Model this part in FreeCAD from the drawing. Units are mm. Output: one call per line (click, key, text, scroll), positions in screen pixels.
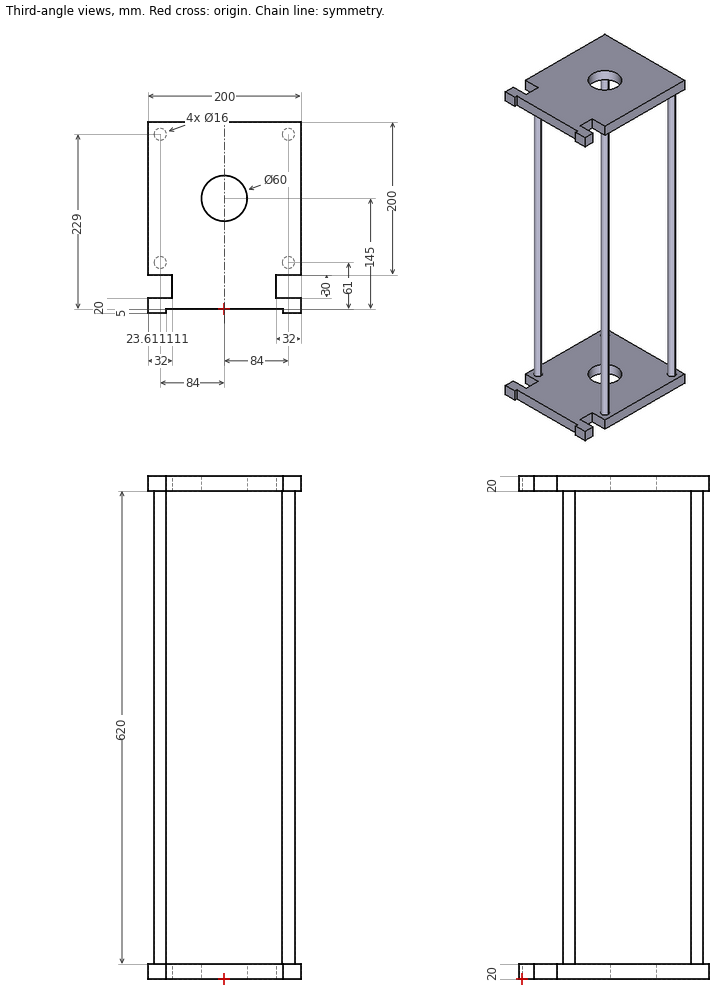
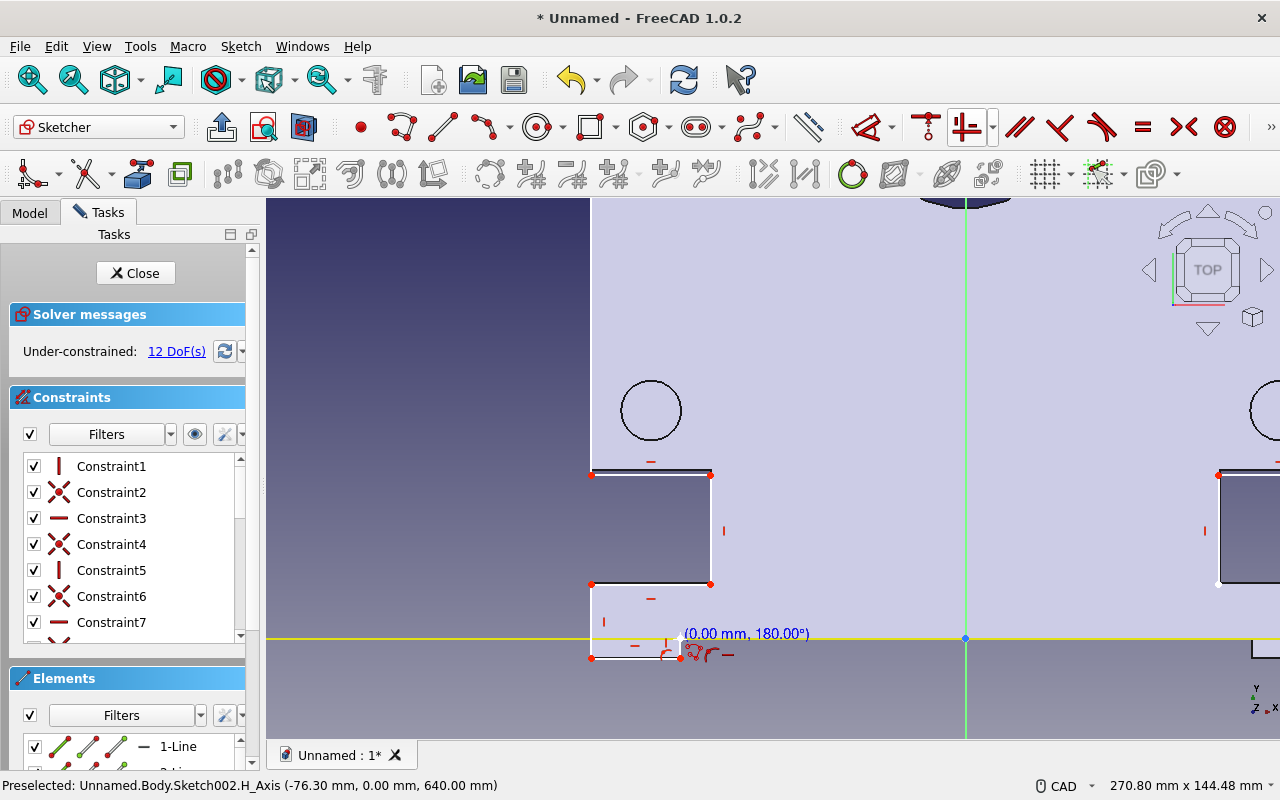
scroll(552, 631, down, 5)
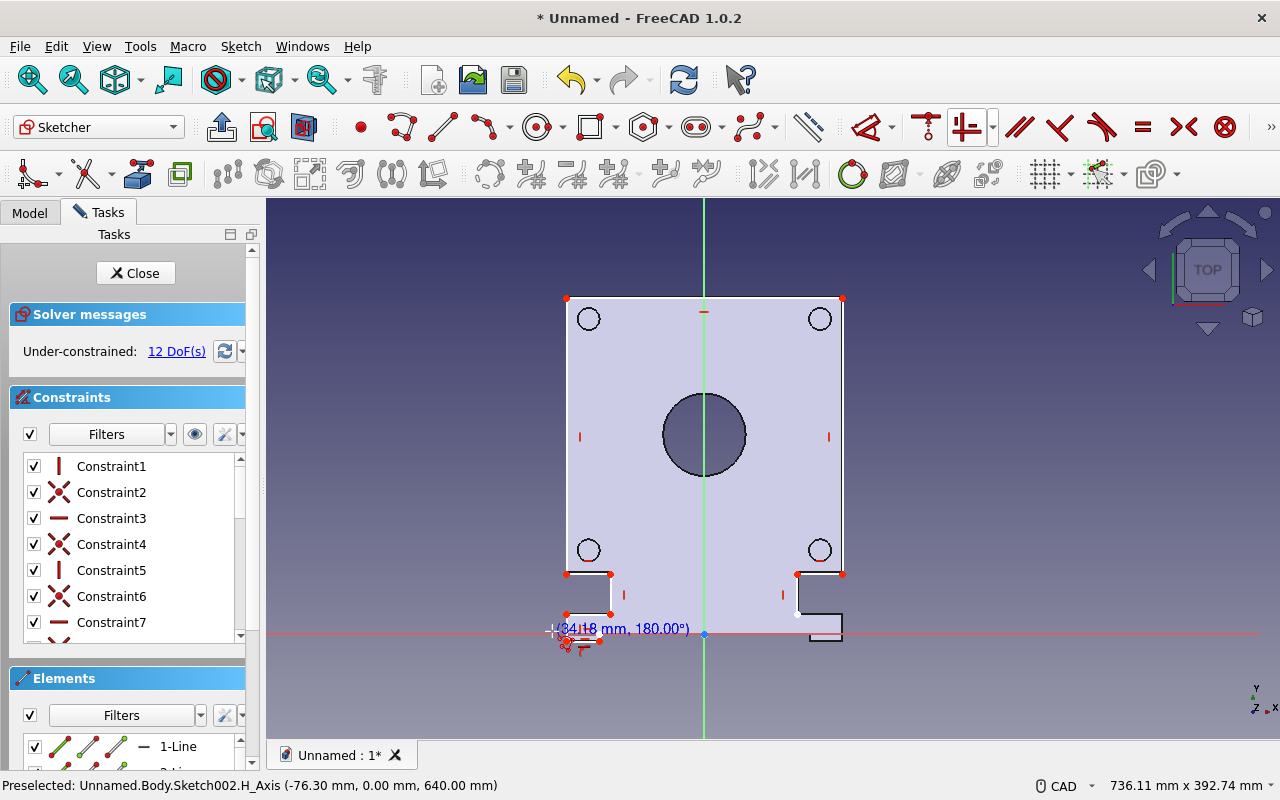
click(810, 625)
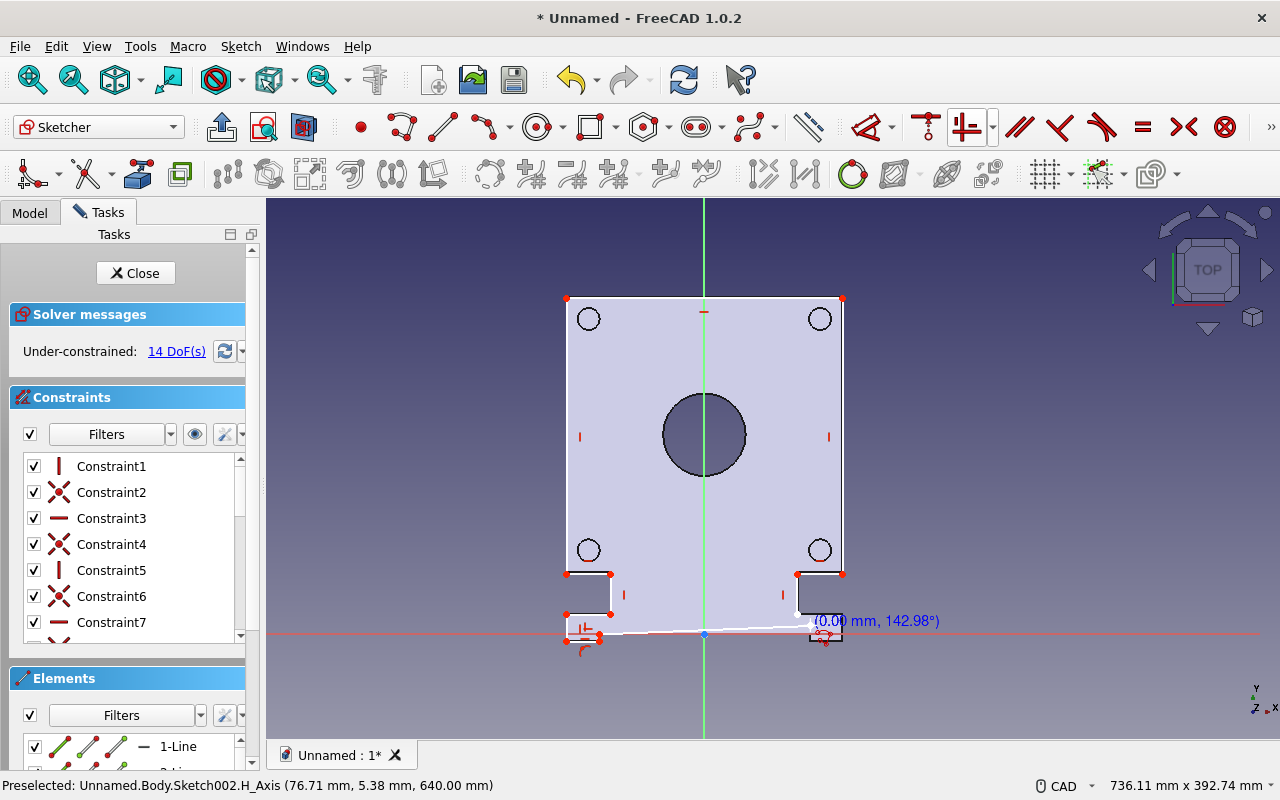
scroll(810, 641, up, 5)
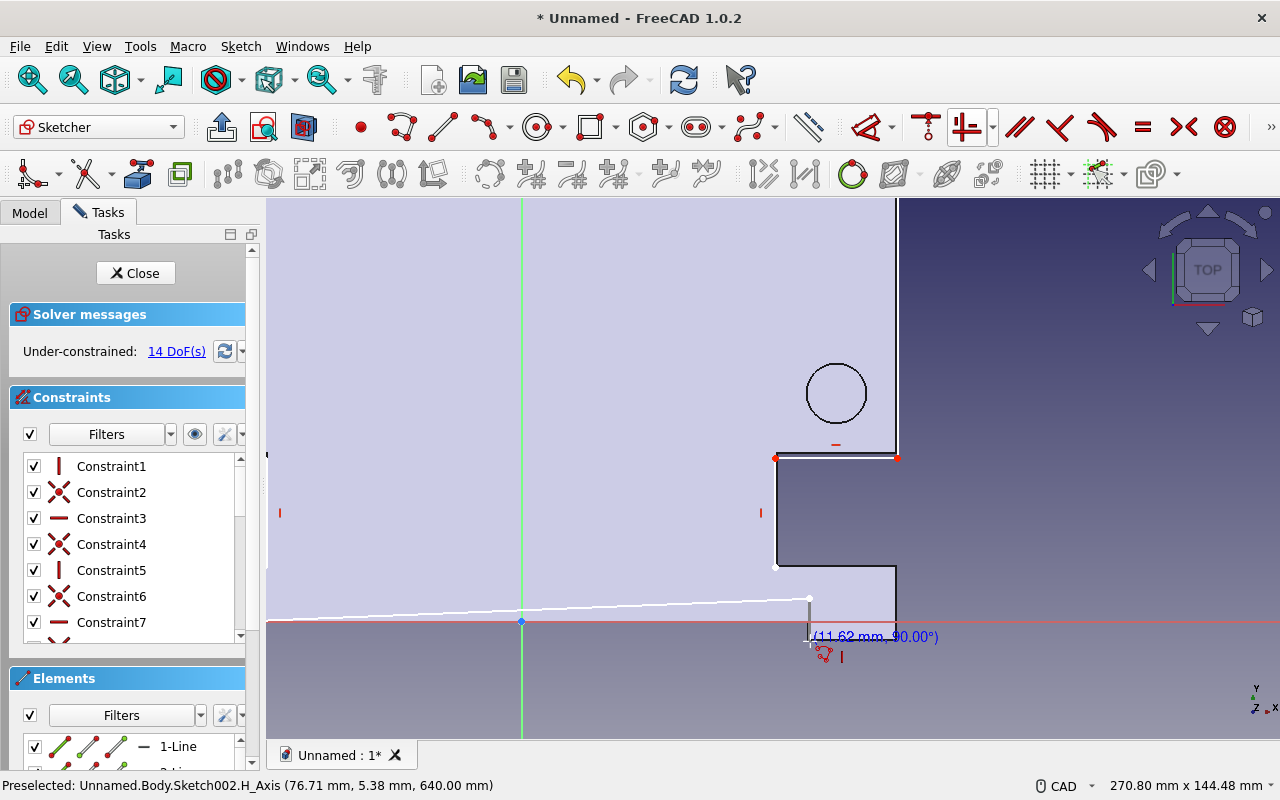
click(809, 640)
click(896, 640)
click(896, 566)
click(775, 568)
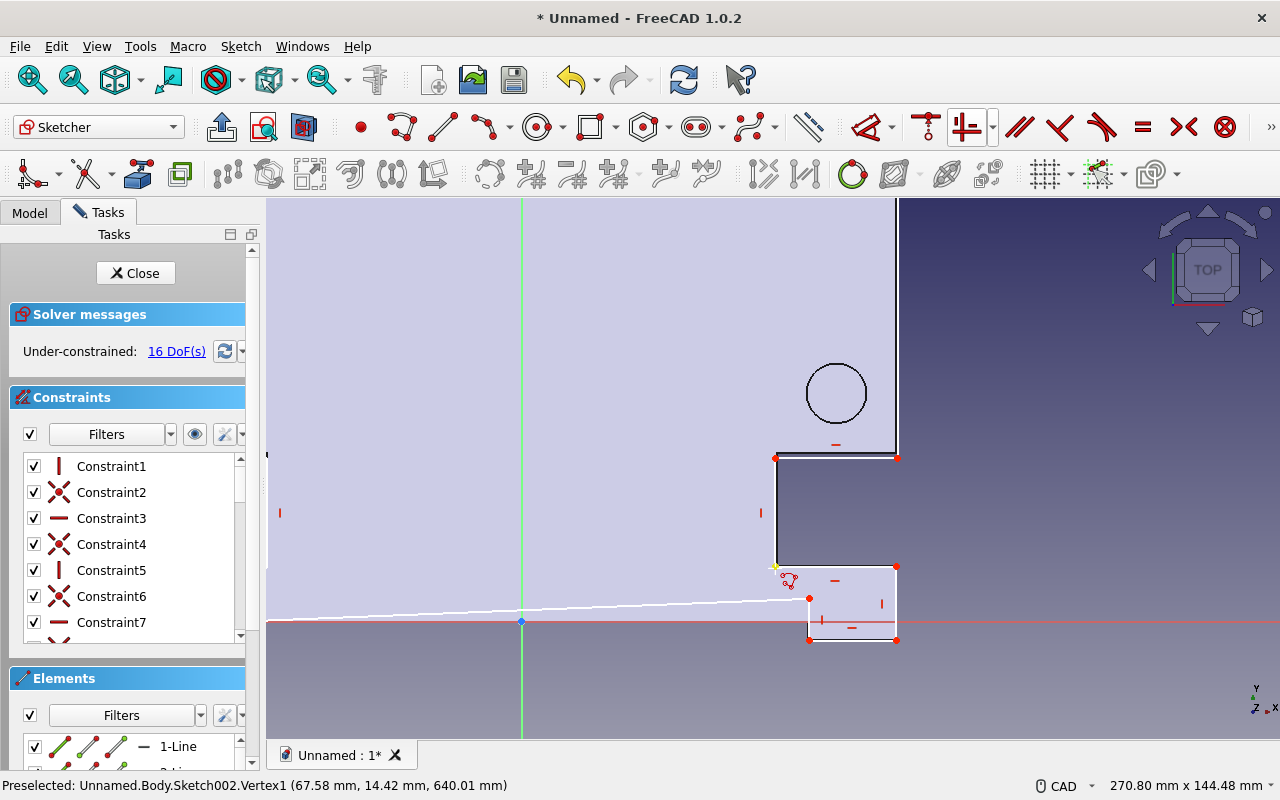
click(536, 128)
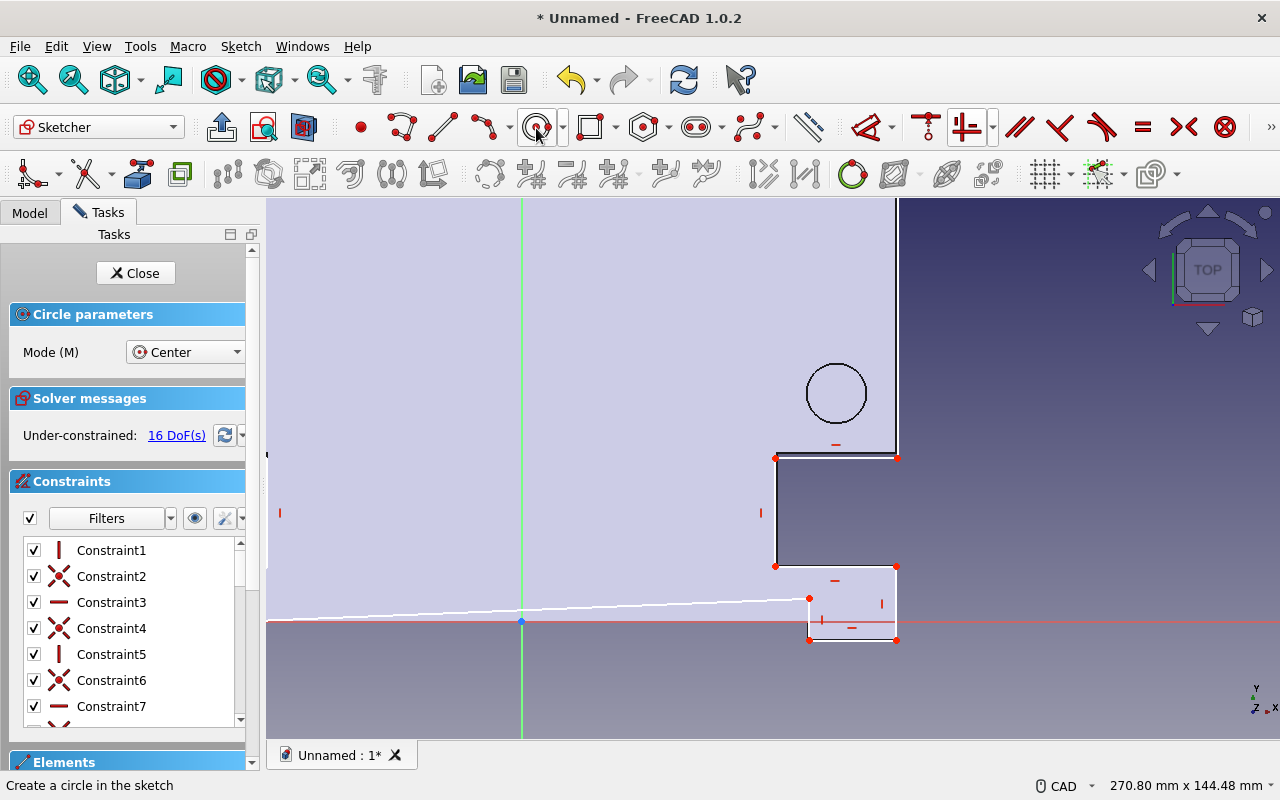
scroll(811, 641, down, 5)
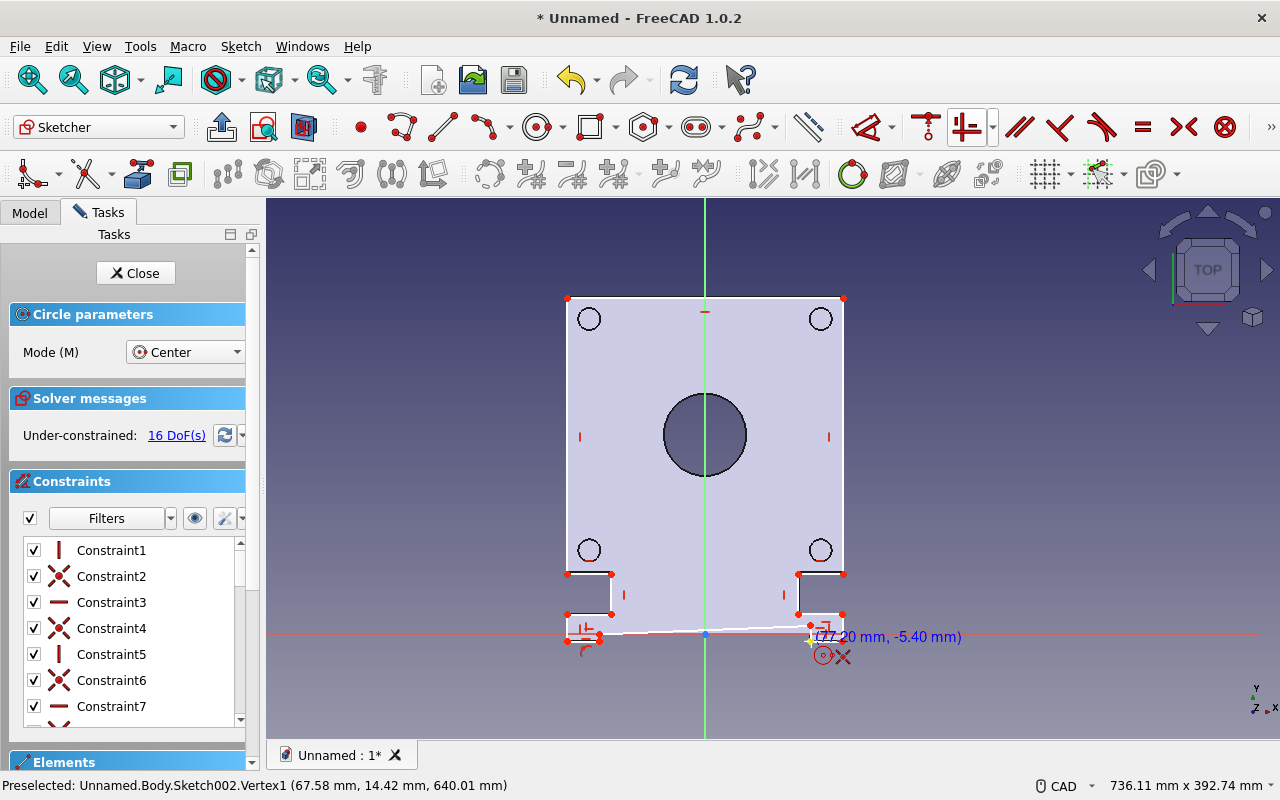
click(705, 435)
click(734, 405)
key(Escape)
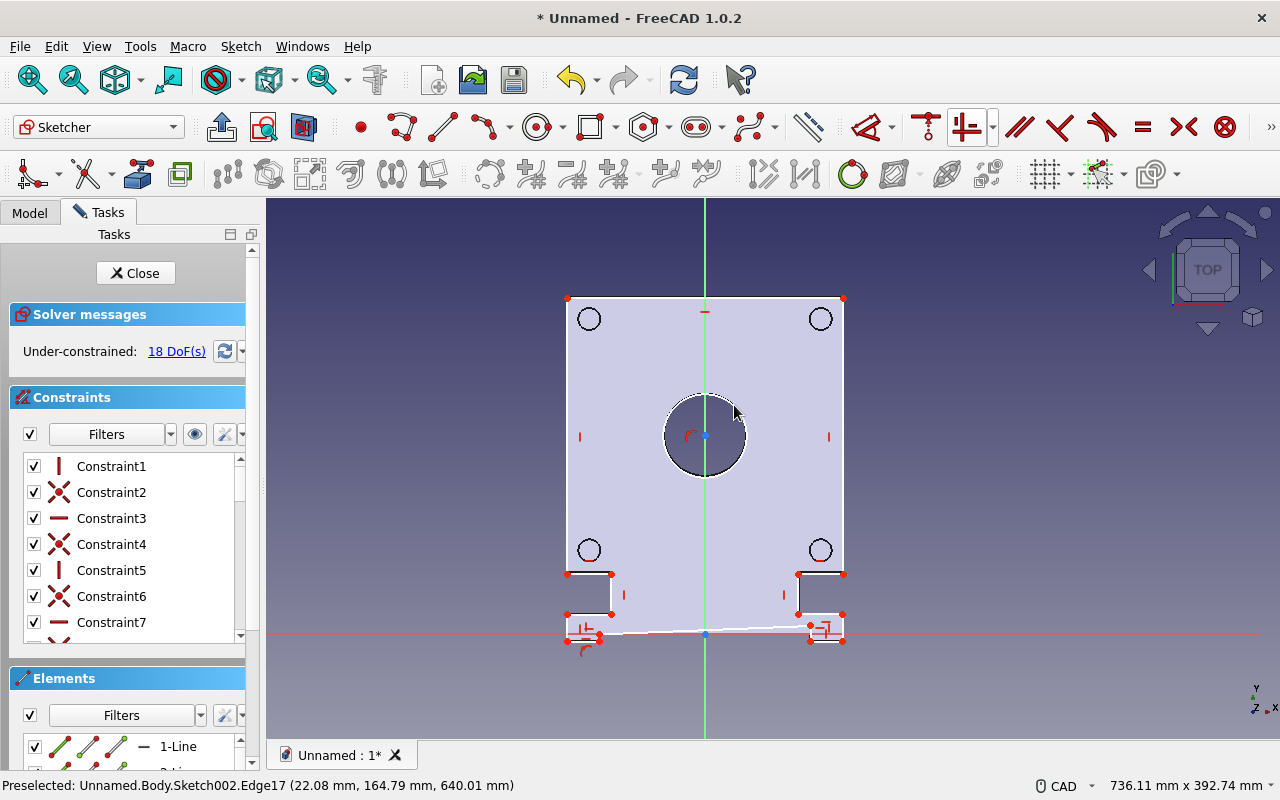
click(663, 632)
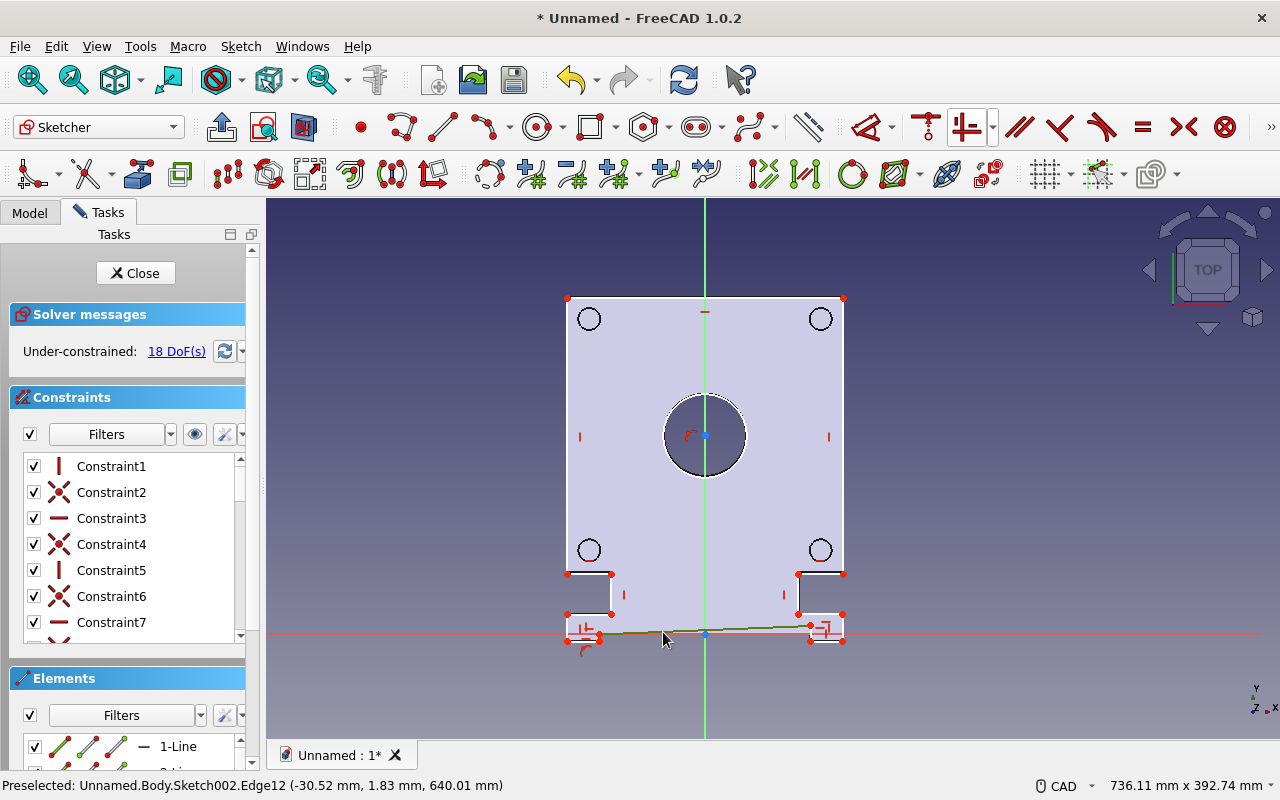
click(992, 128)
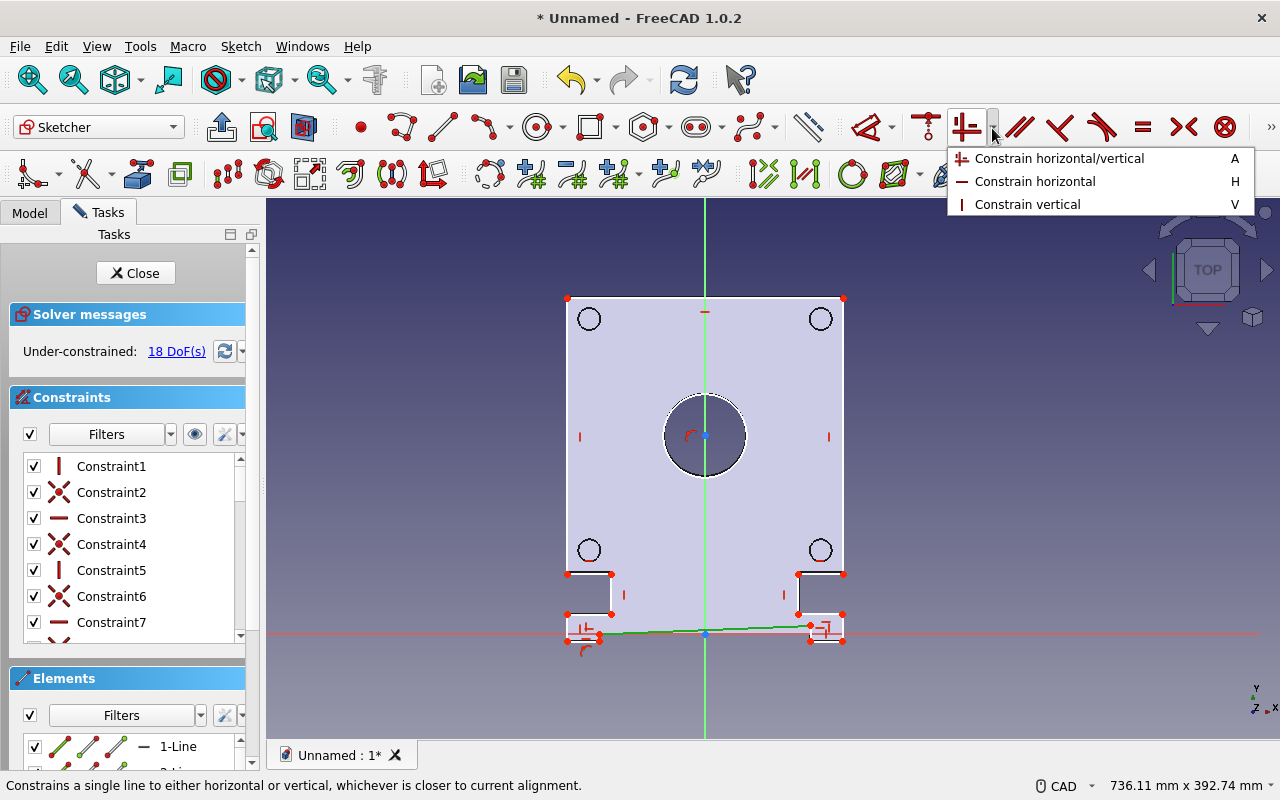
click(1101, 182)